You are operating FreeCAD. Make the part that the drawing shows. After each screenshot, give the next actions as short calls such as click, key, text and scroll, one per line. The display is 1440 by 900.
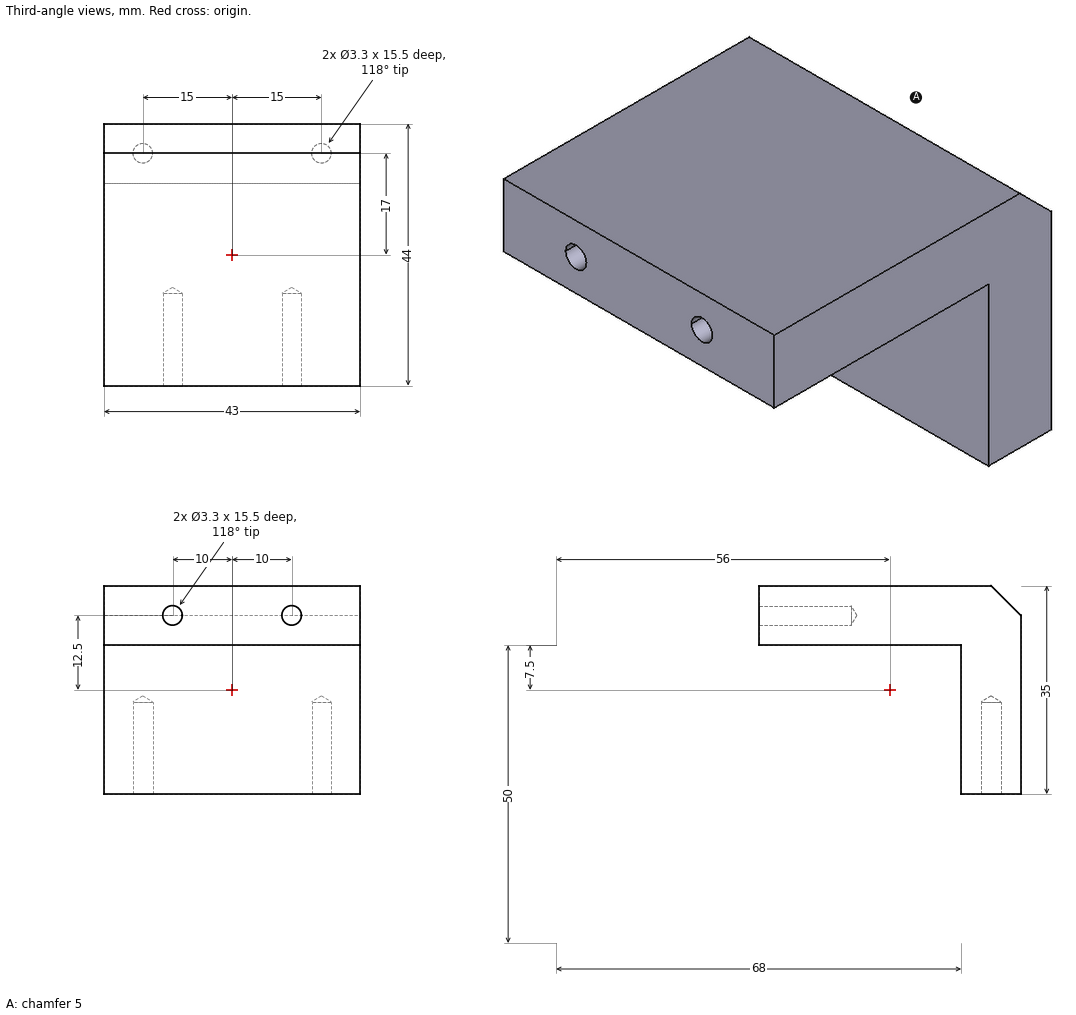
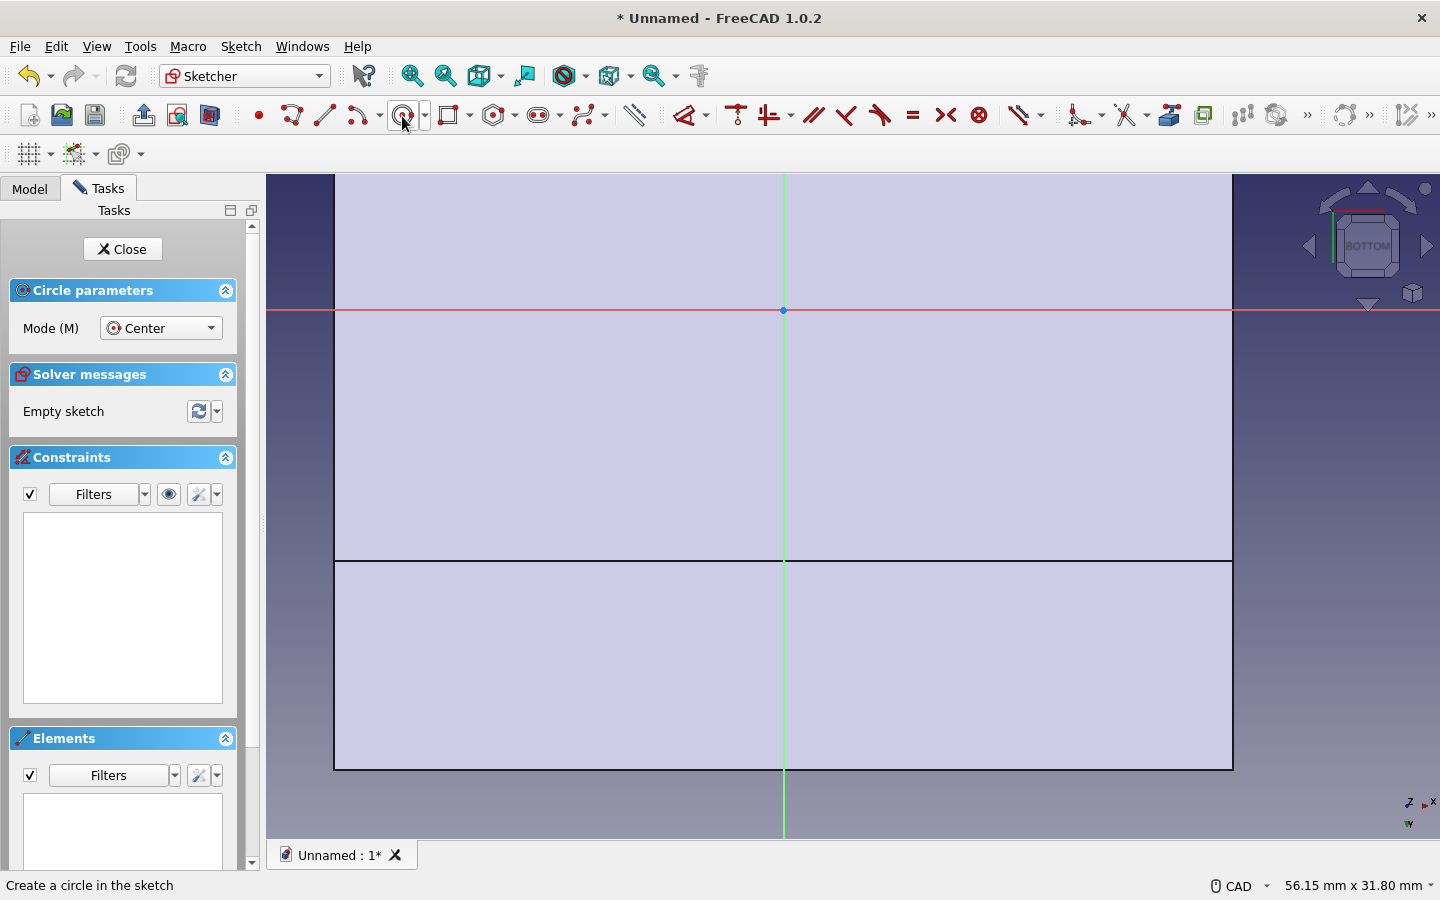
click(1097, 666)
click(1122, 641)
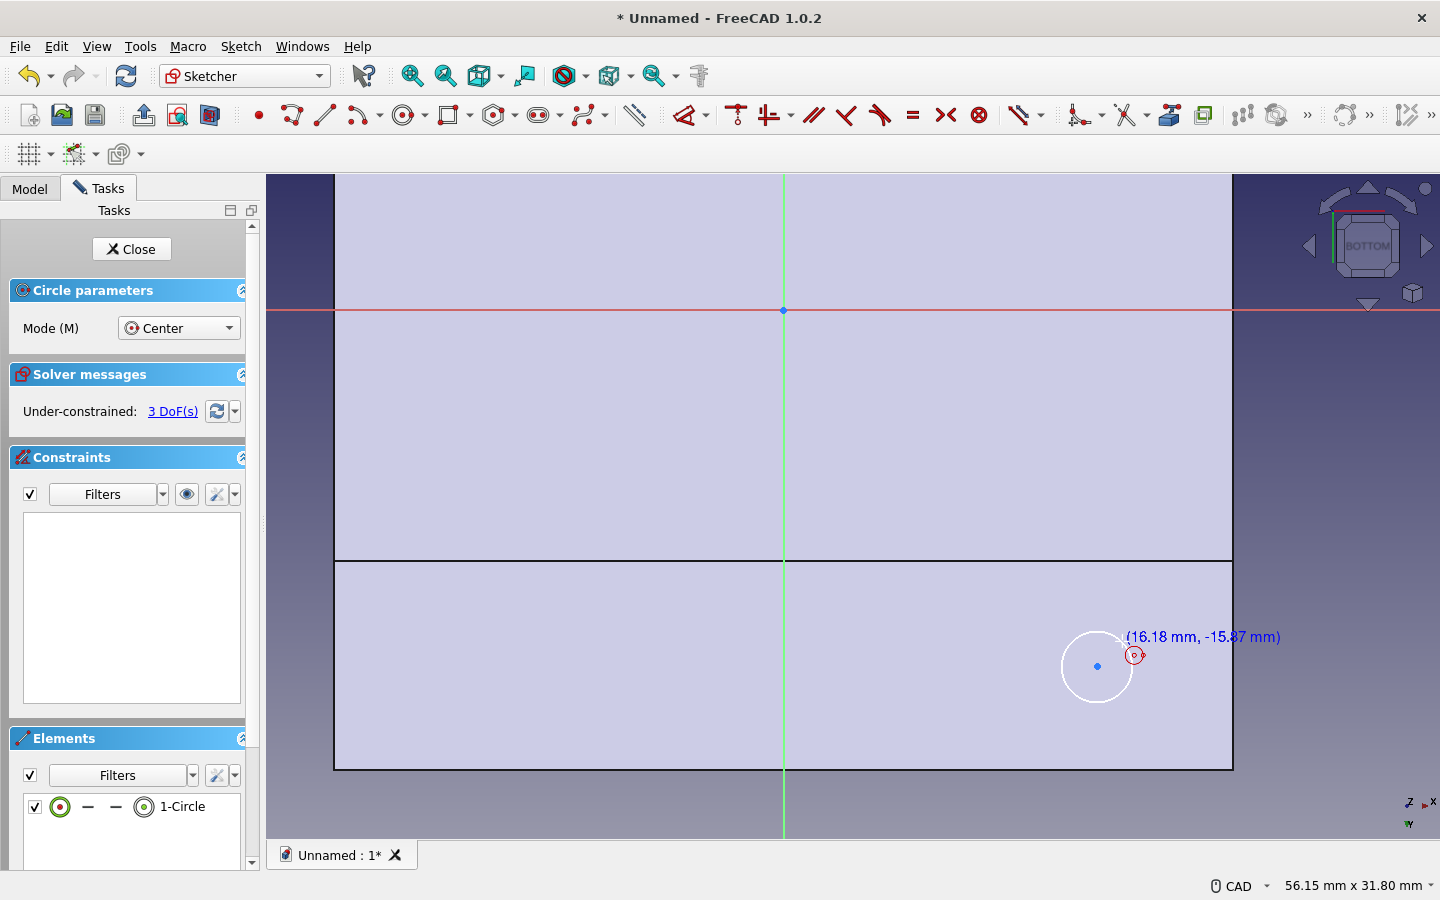
click(470, 666)
click(494, 641)
key(Escape)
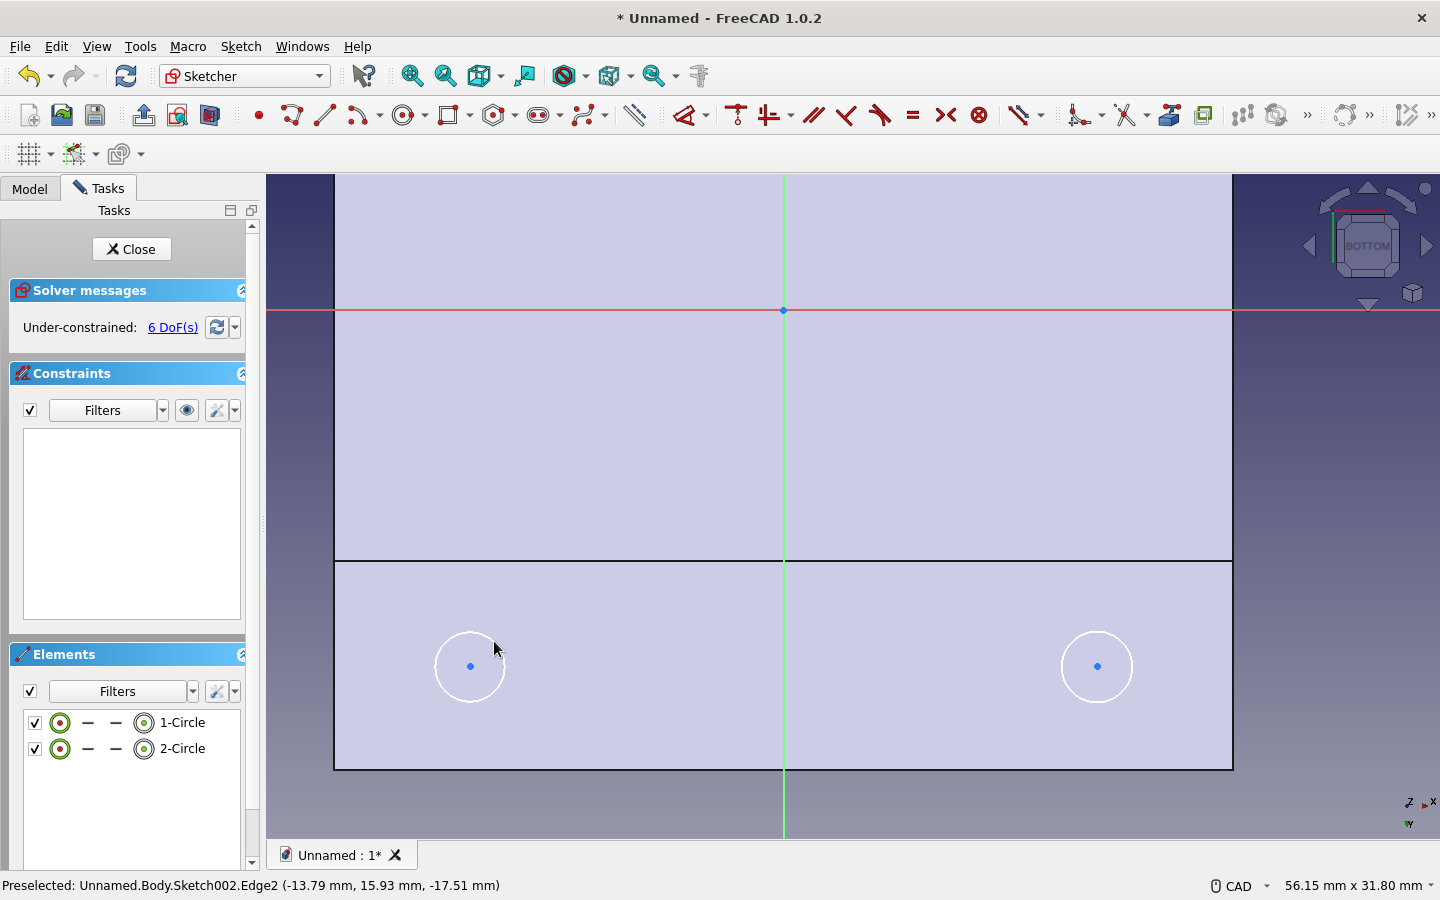
click(1122, 642)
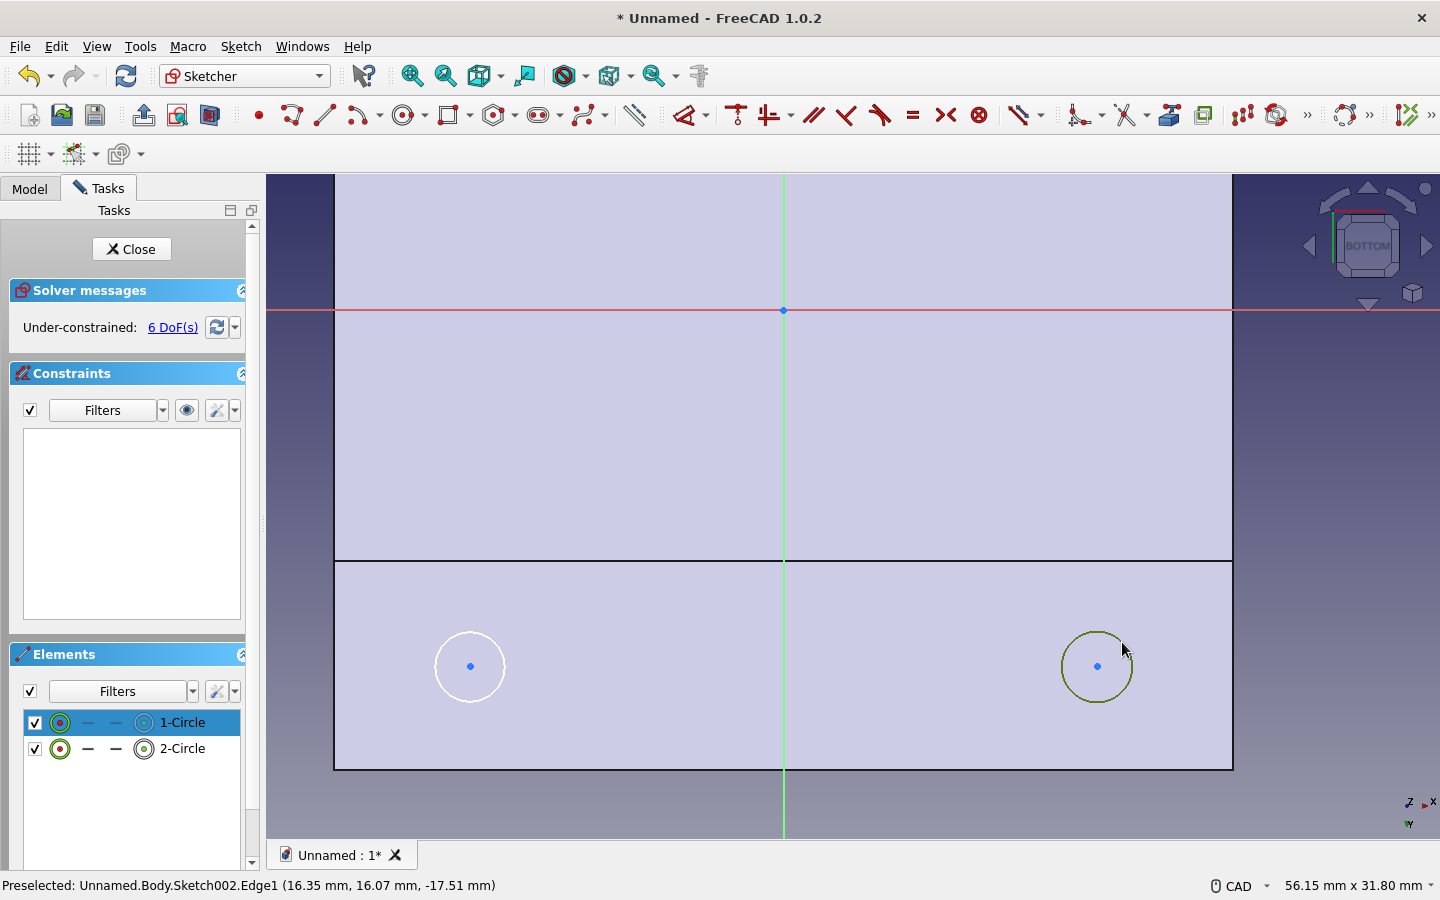
click(494, 642)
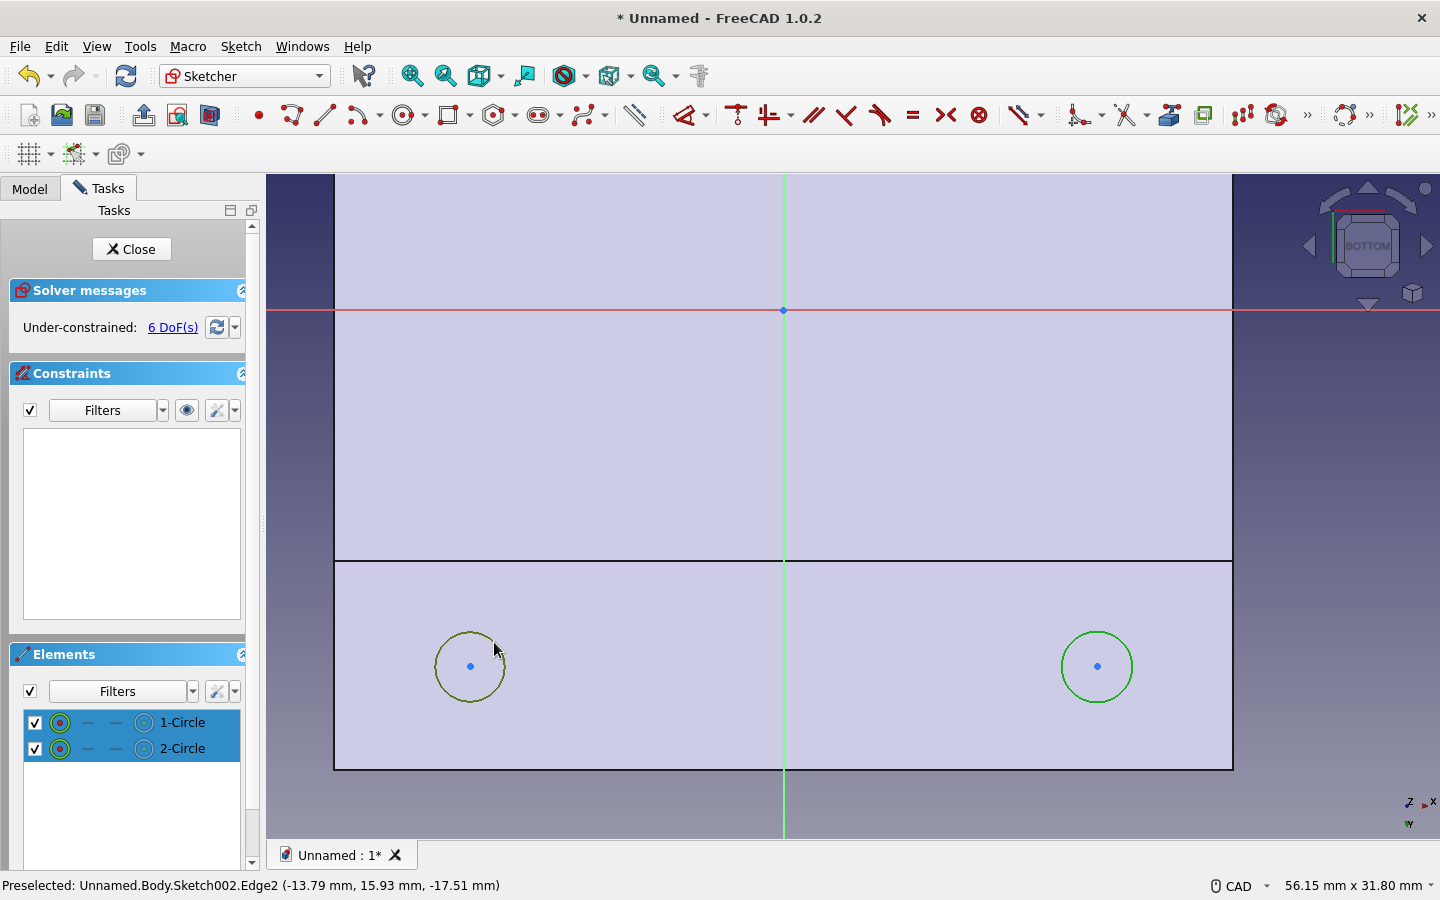
click(913, 116)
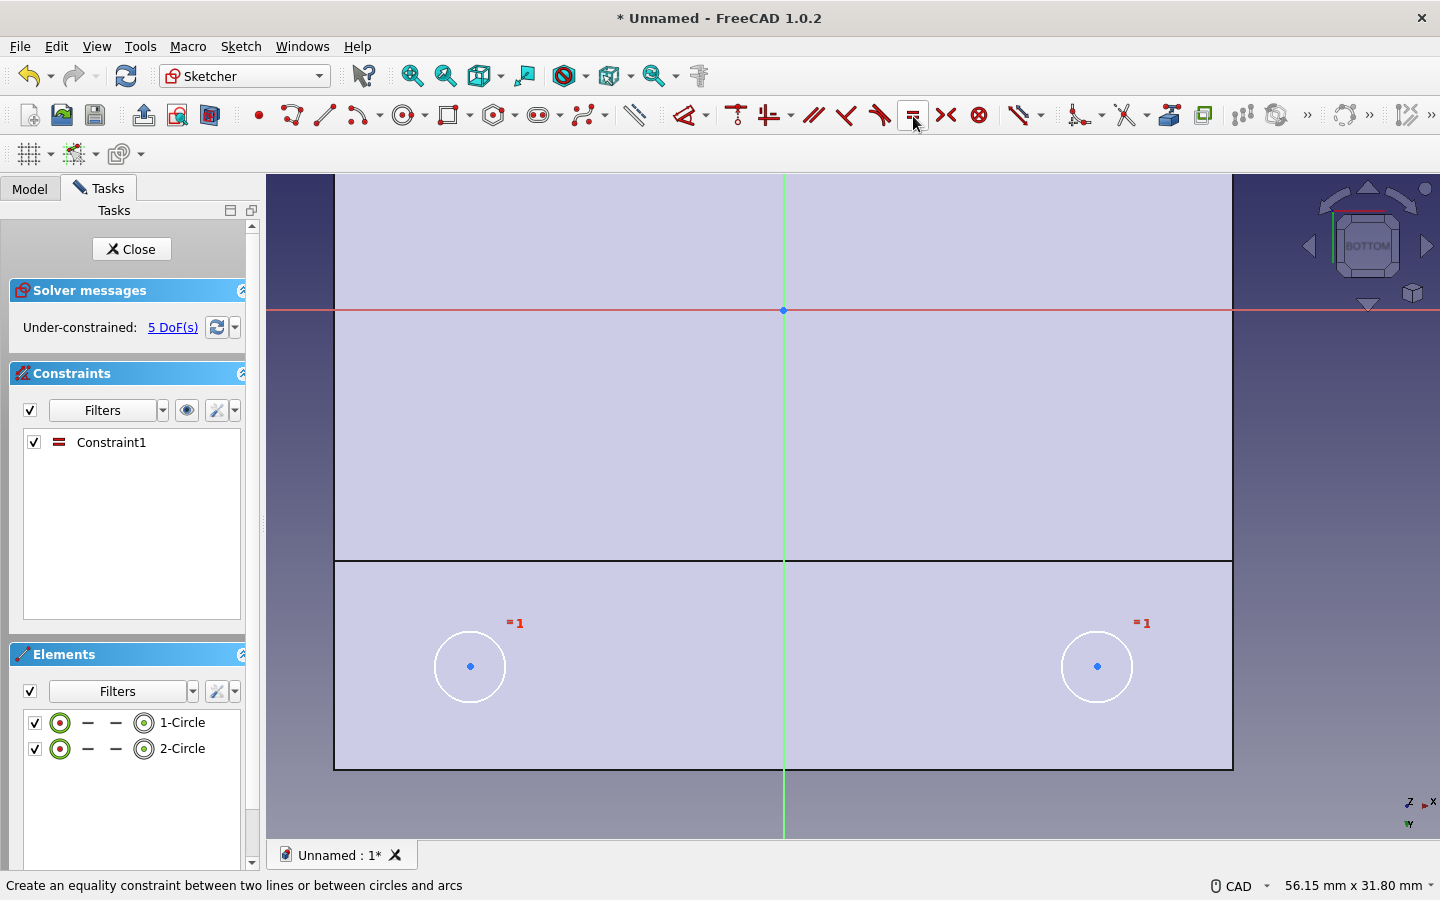
click(684, 116)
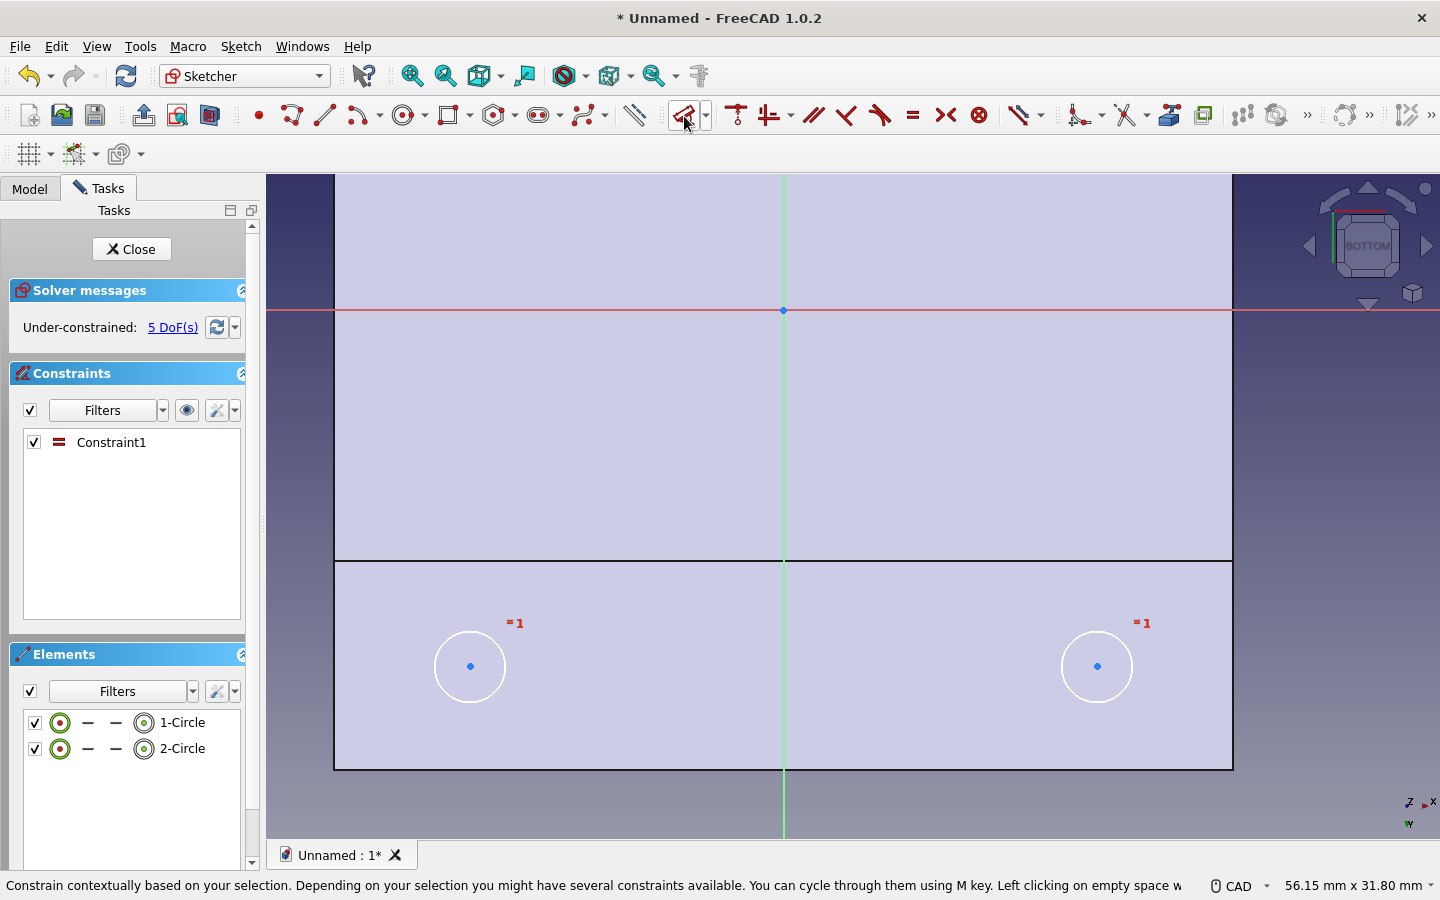
click(1122, 642)
click(1145, 619)